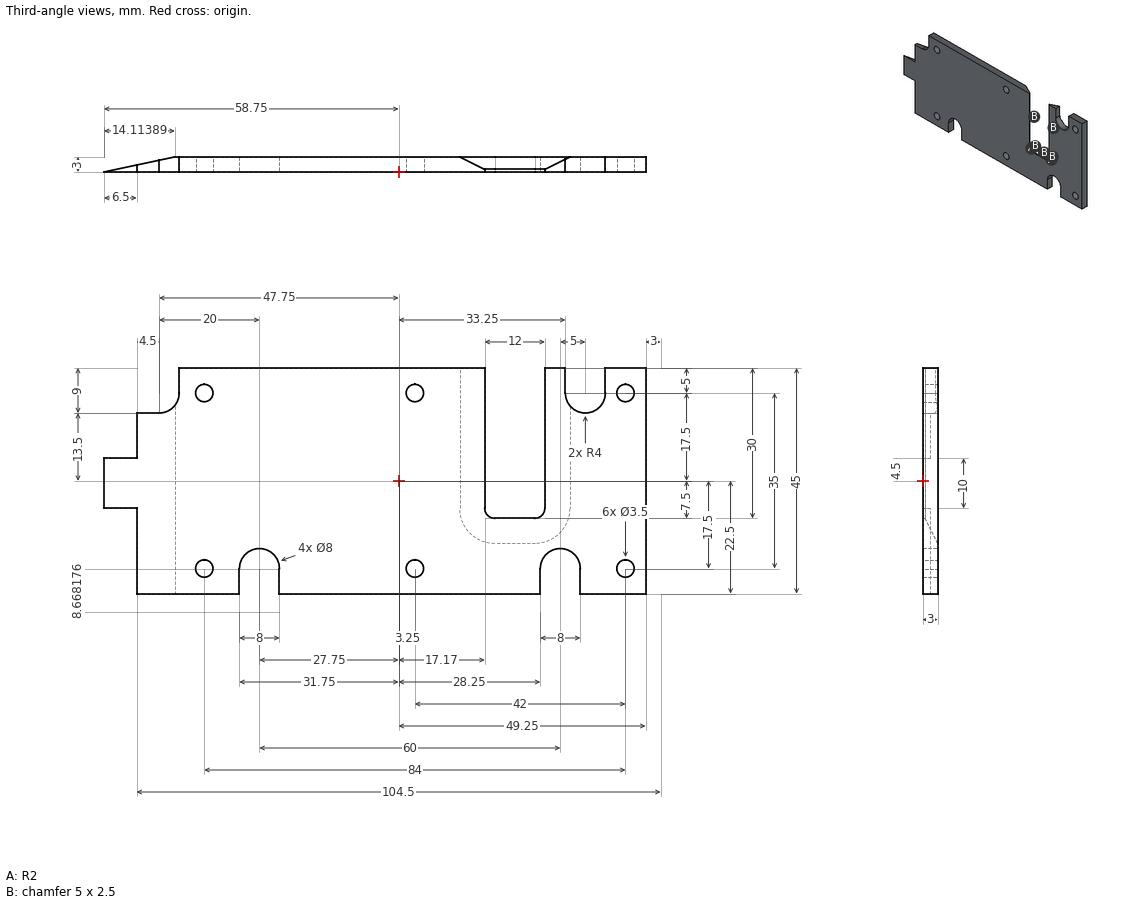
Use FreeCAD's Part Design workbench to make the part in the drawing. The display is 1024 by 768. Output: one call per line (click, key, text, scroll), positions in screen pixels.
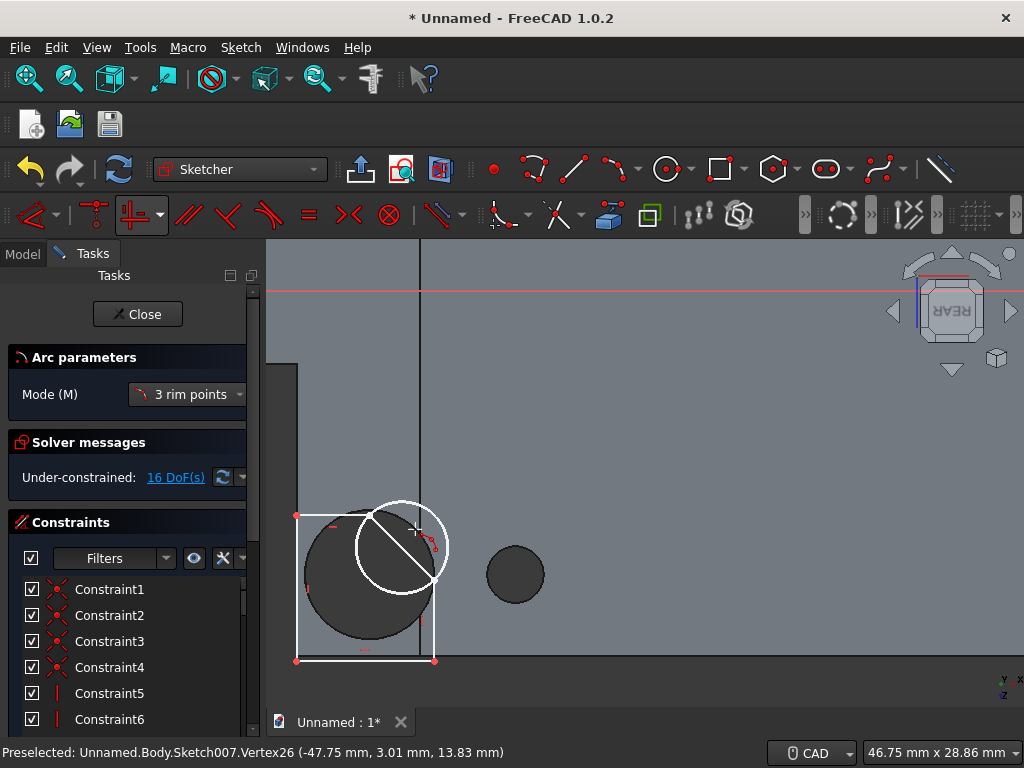
click(415, 529)
key(Escape)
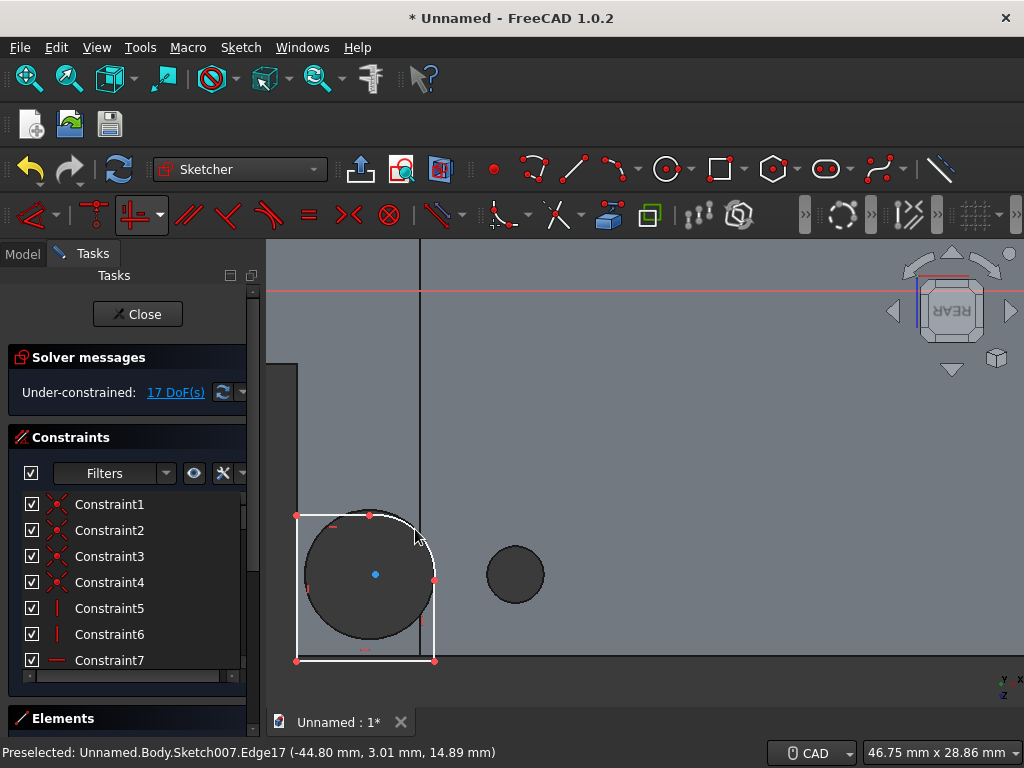
scroll(420, 542, down, 7)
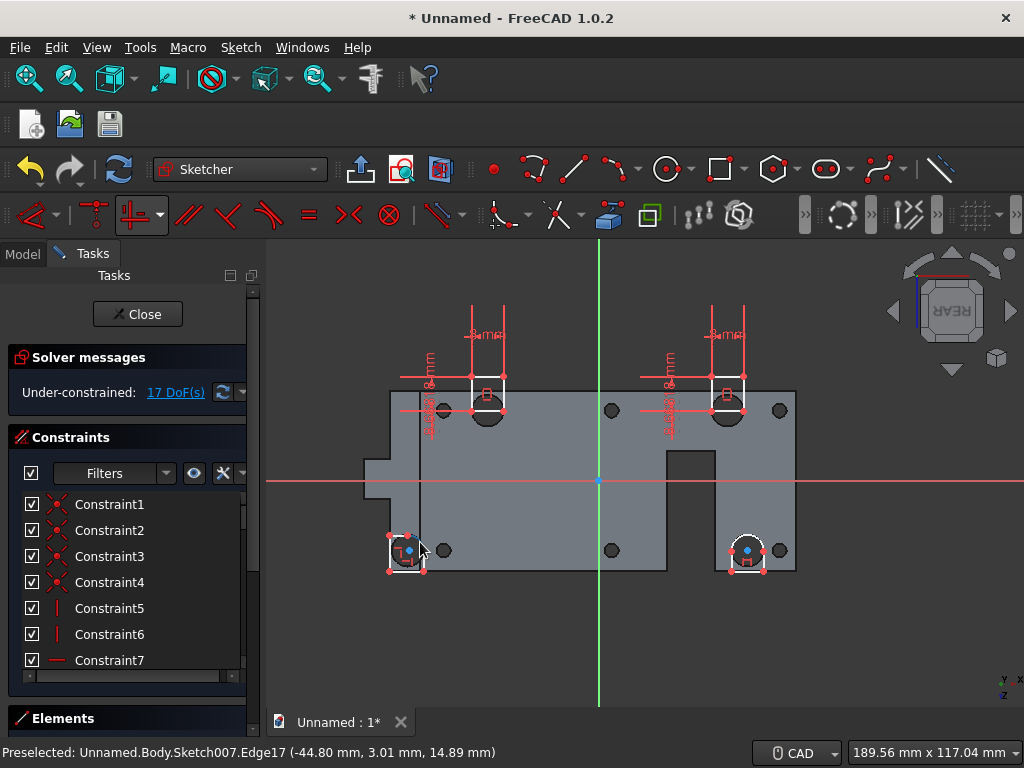
scroll(732, 558, up, 5)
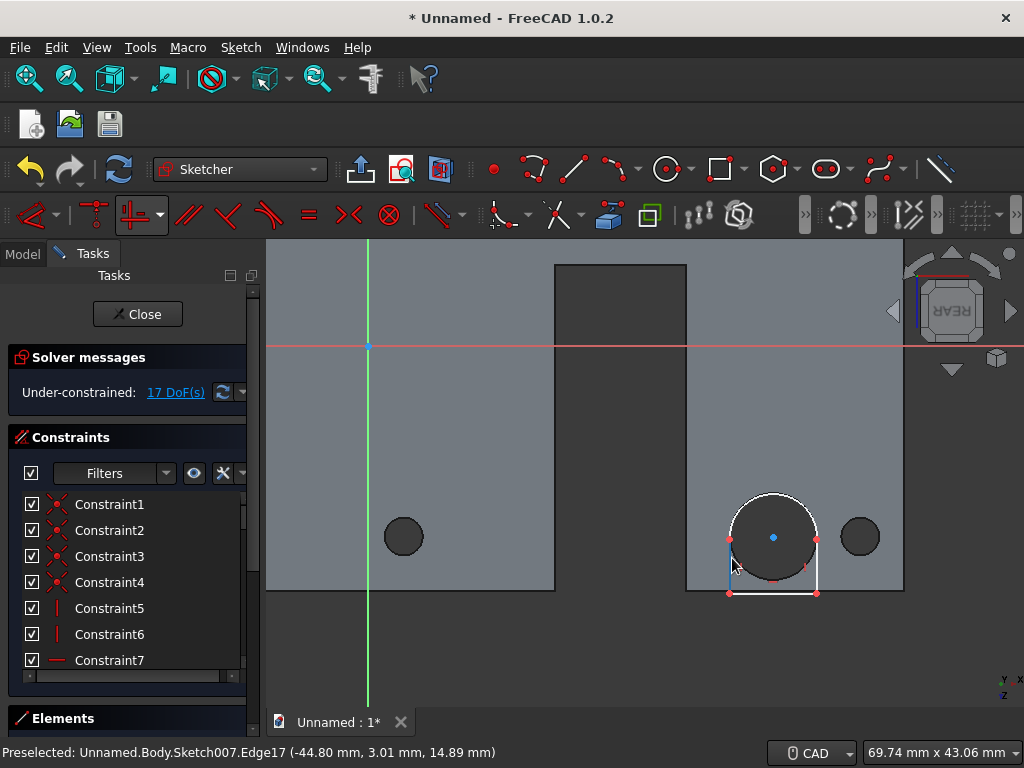
click(730, 556)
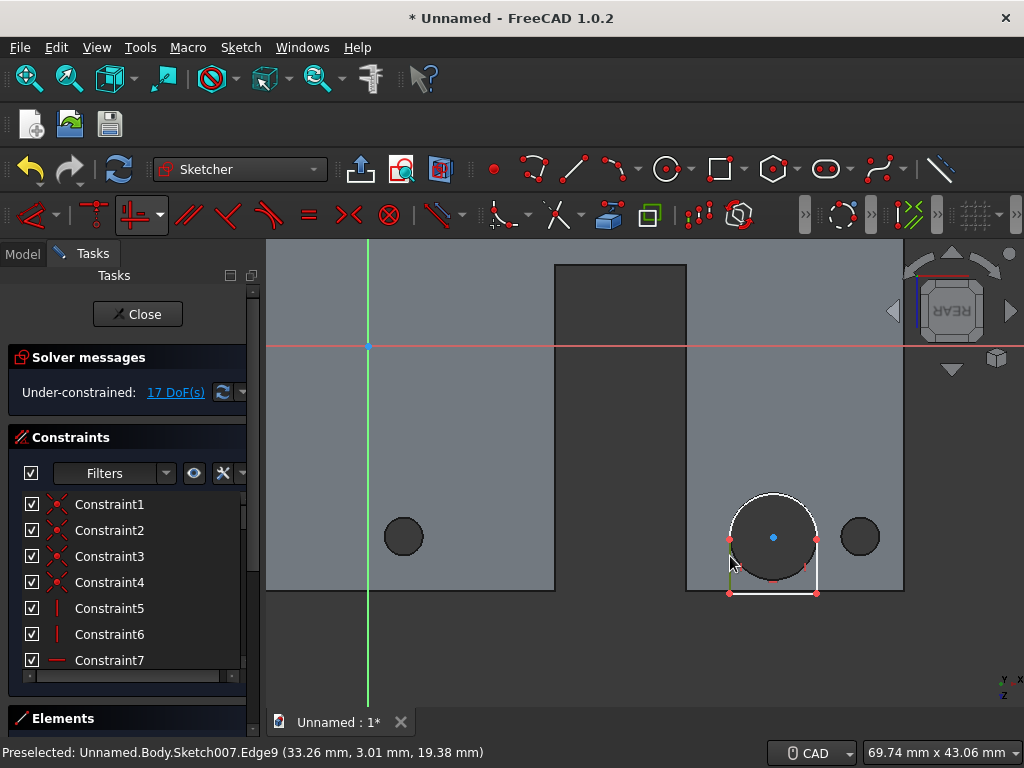
click(800, 503)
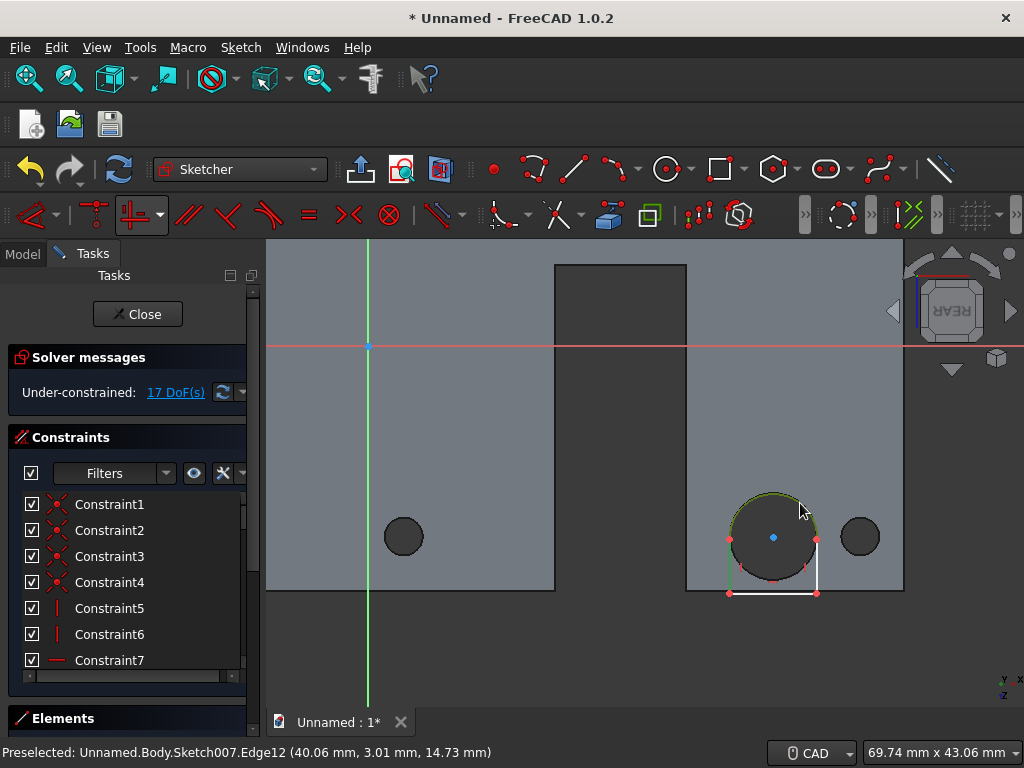
click(270, 216)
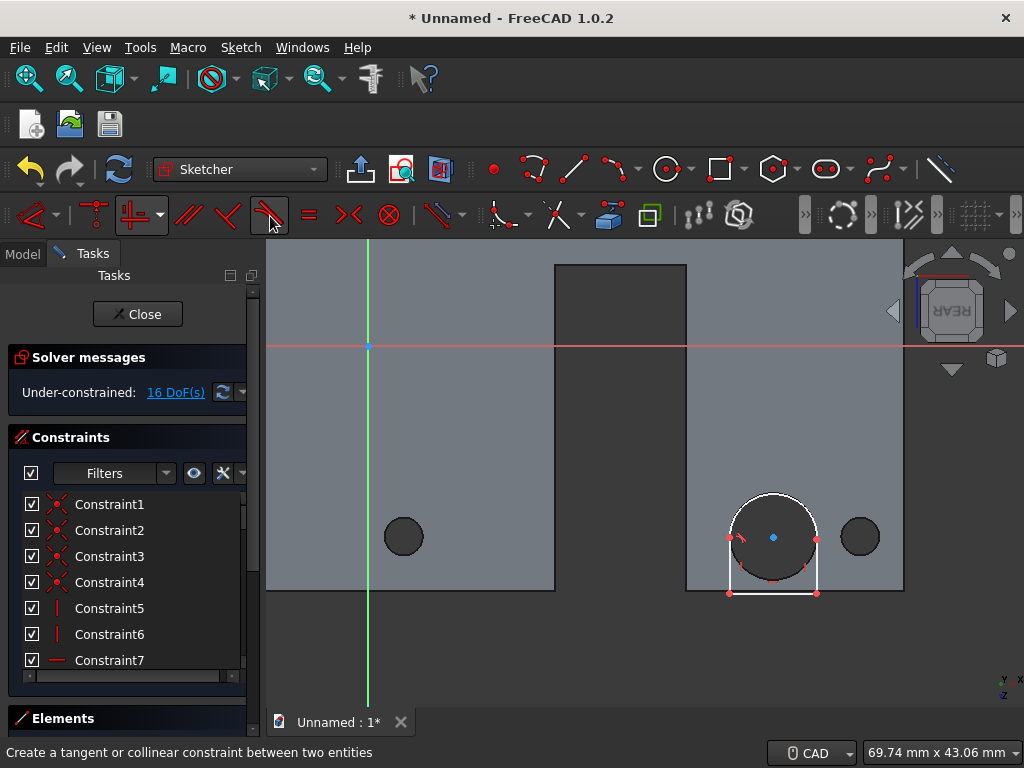
click(817, 577)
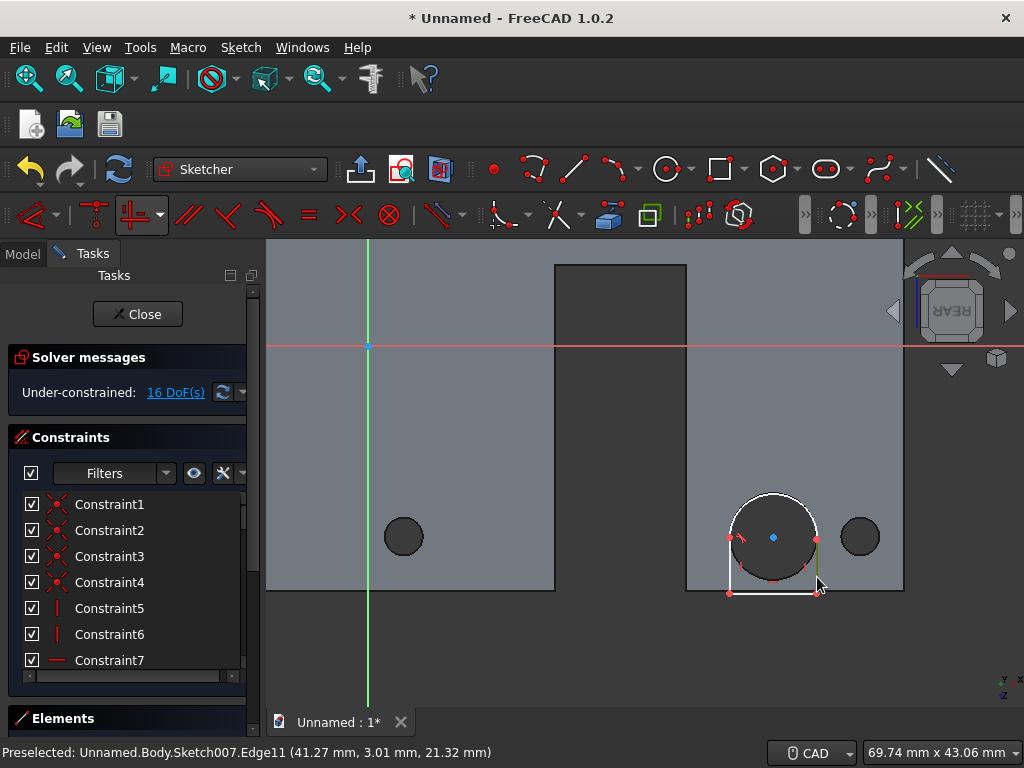
click(800, 503)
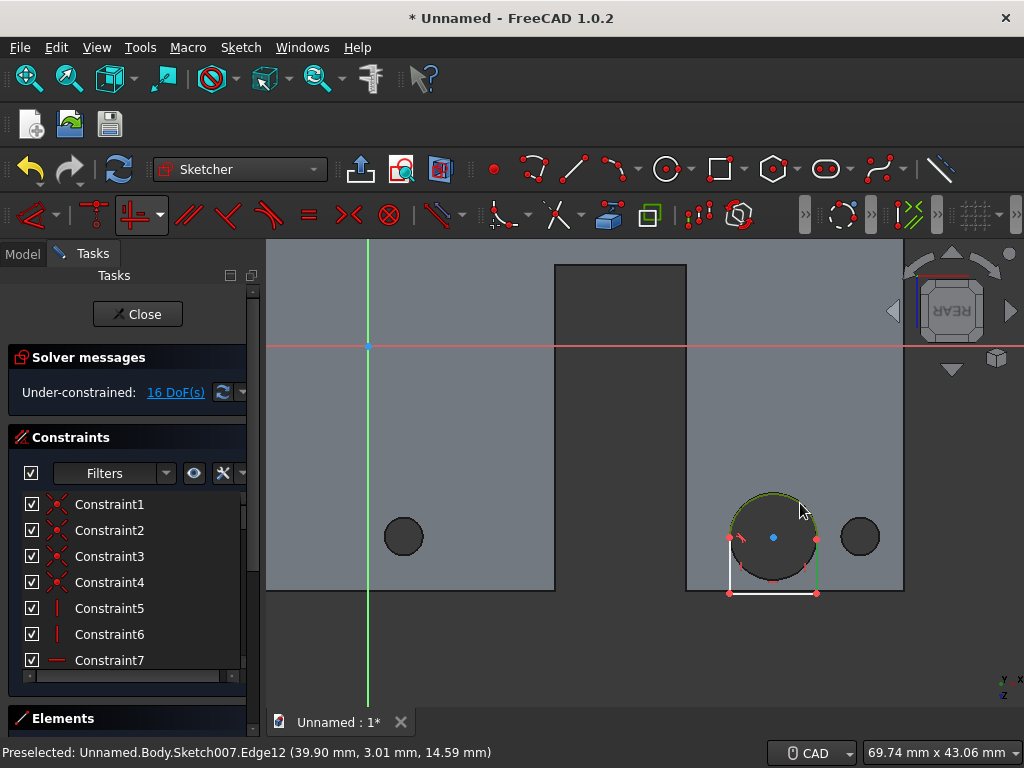
click(270, 216)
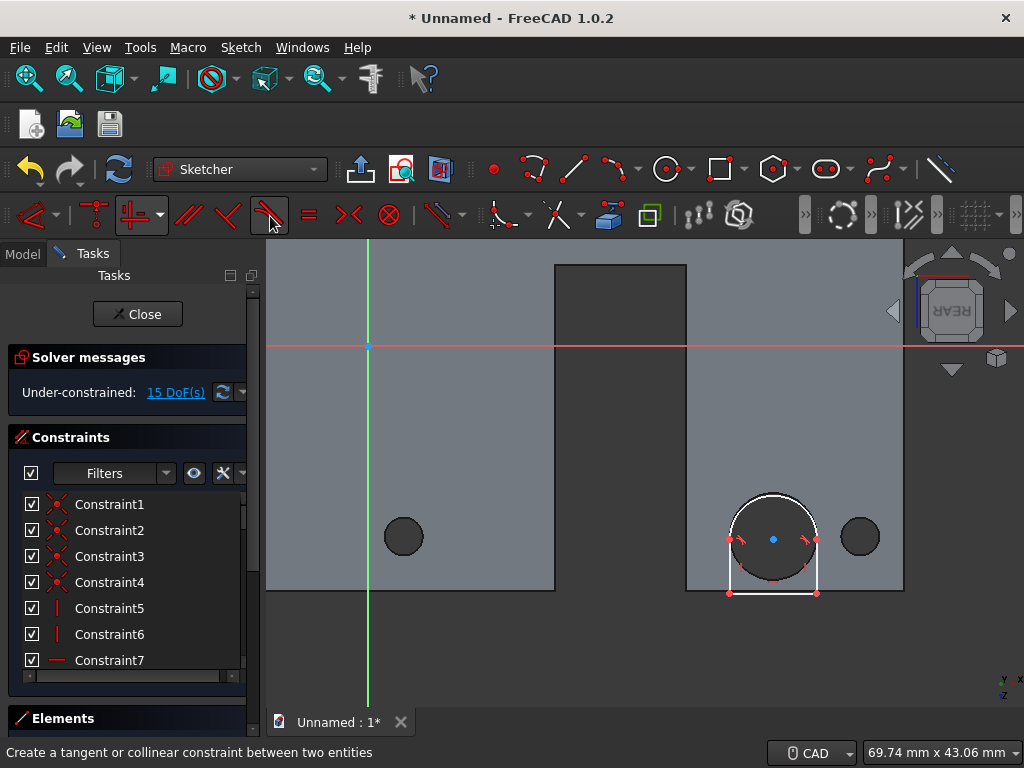
scroll(732, 558, down, 5)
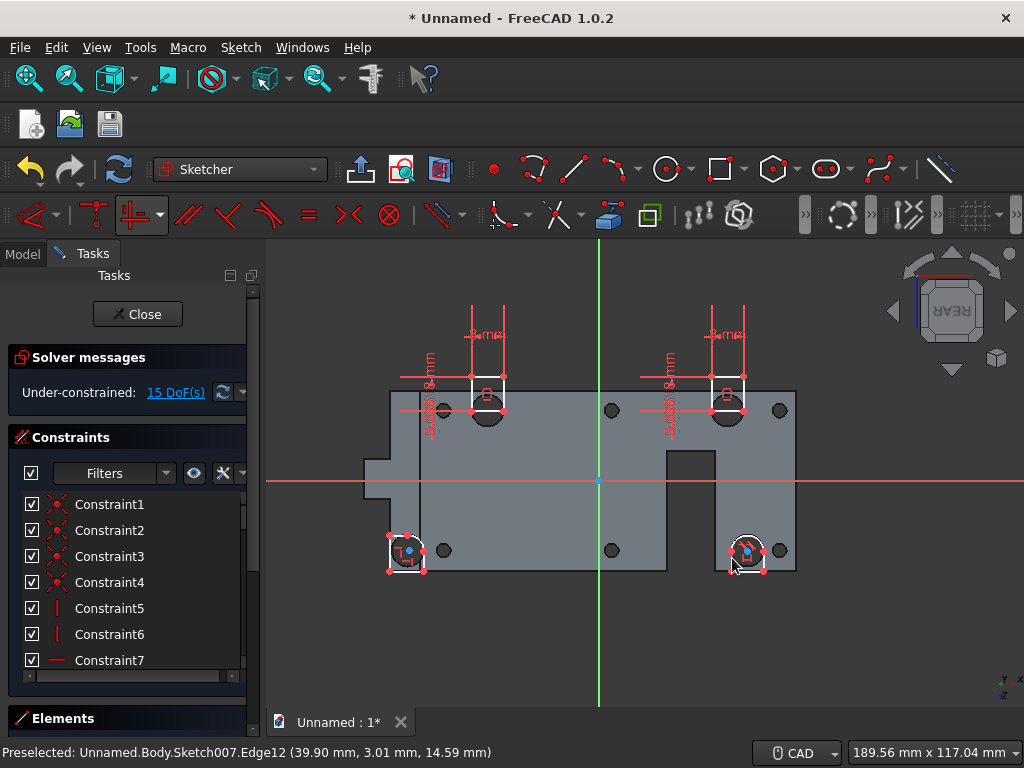
scroll(402, 536, up, 5)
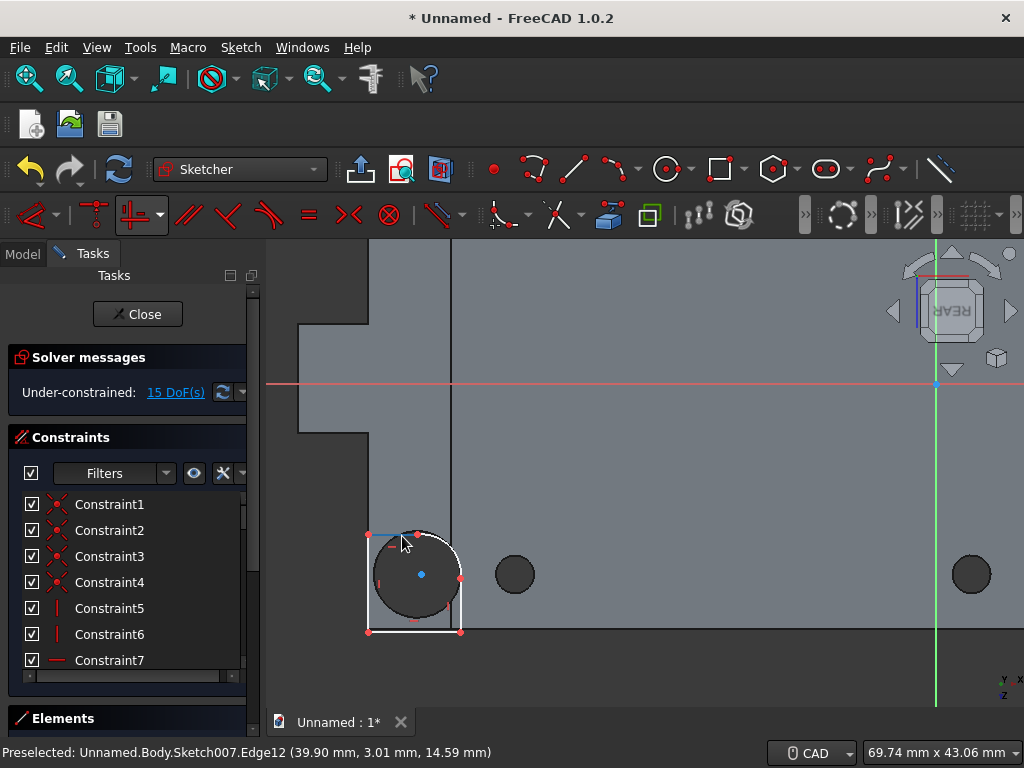
click(403, 535)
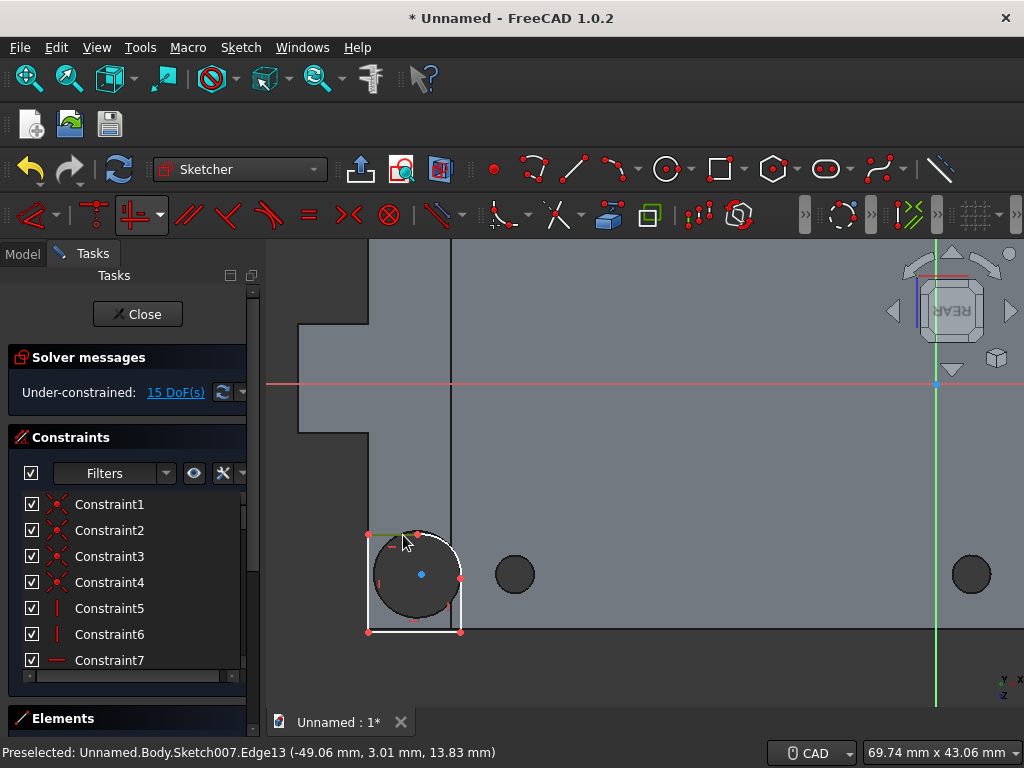
click(457, 557)